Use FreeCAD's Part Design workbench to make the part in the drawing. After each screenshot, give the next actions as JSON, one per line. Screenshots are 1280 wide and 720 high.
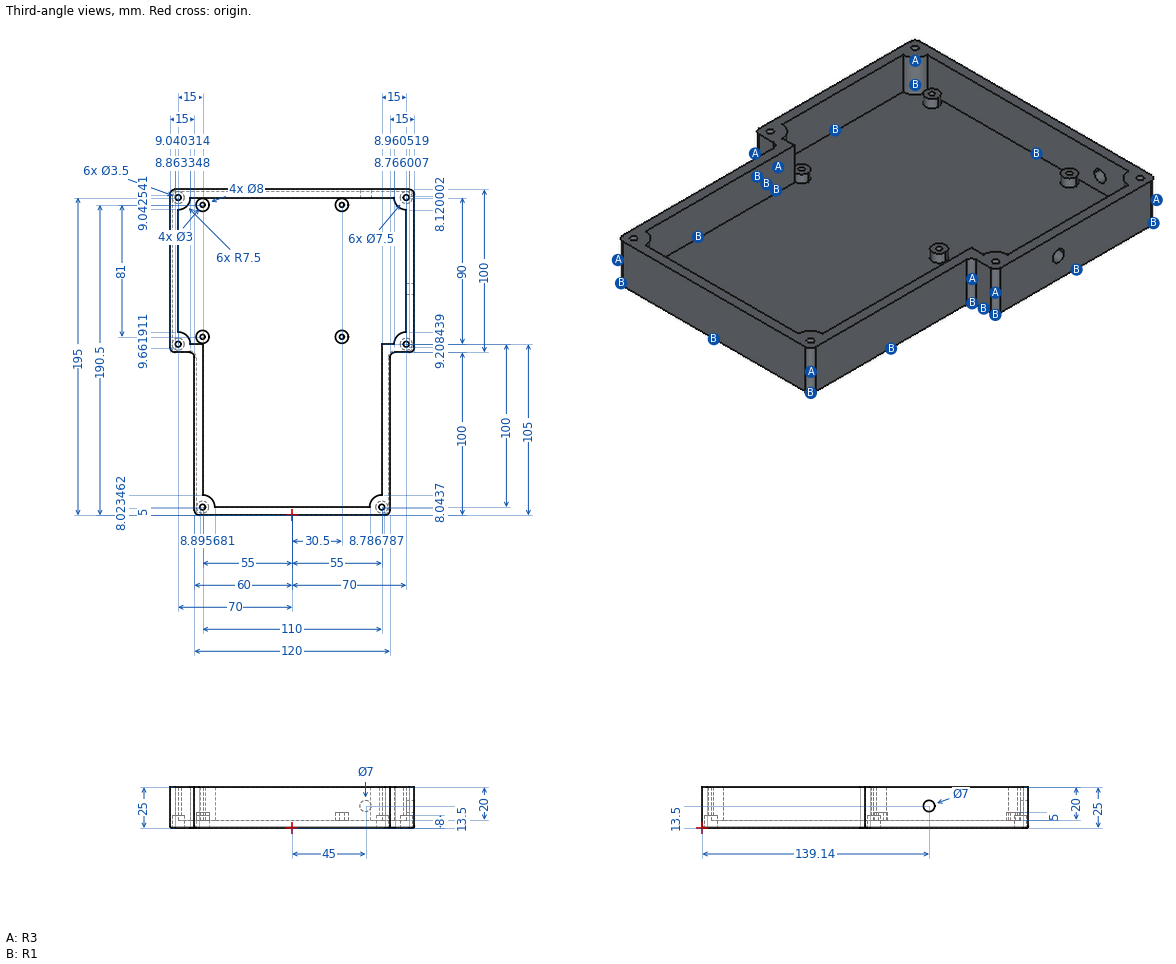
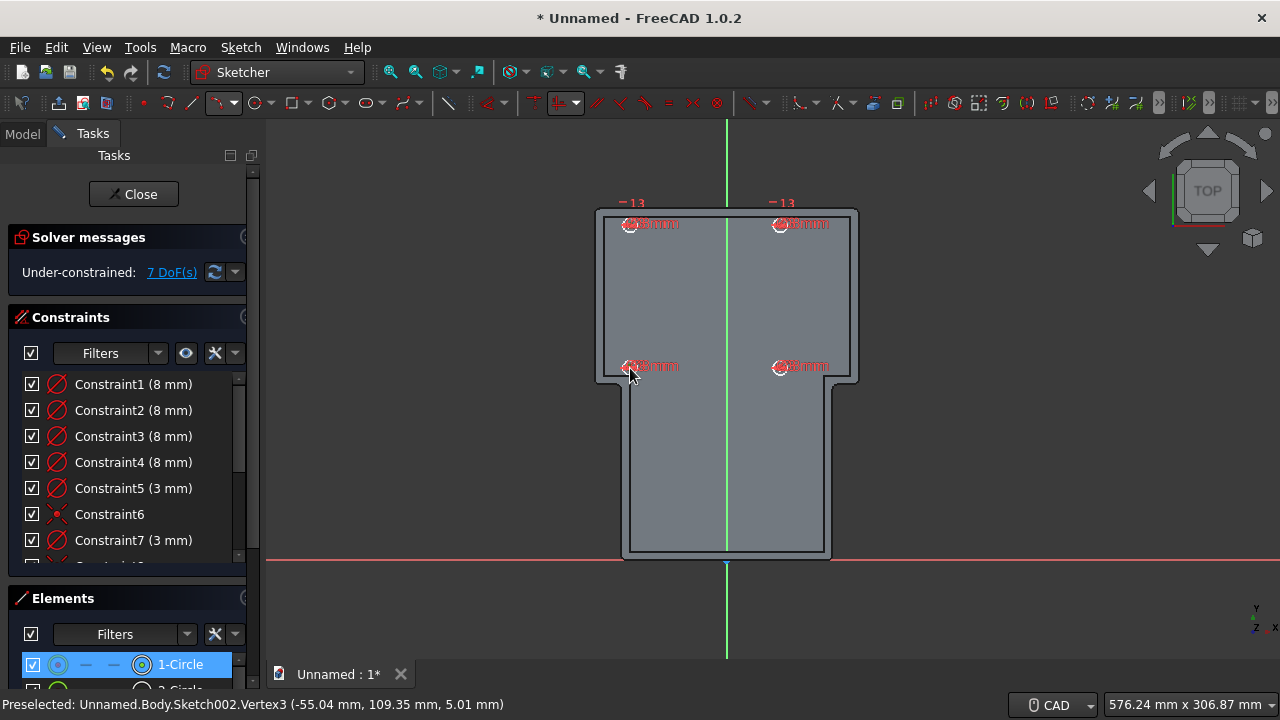
{"action": "key", "text": "v"}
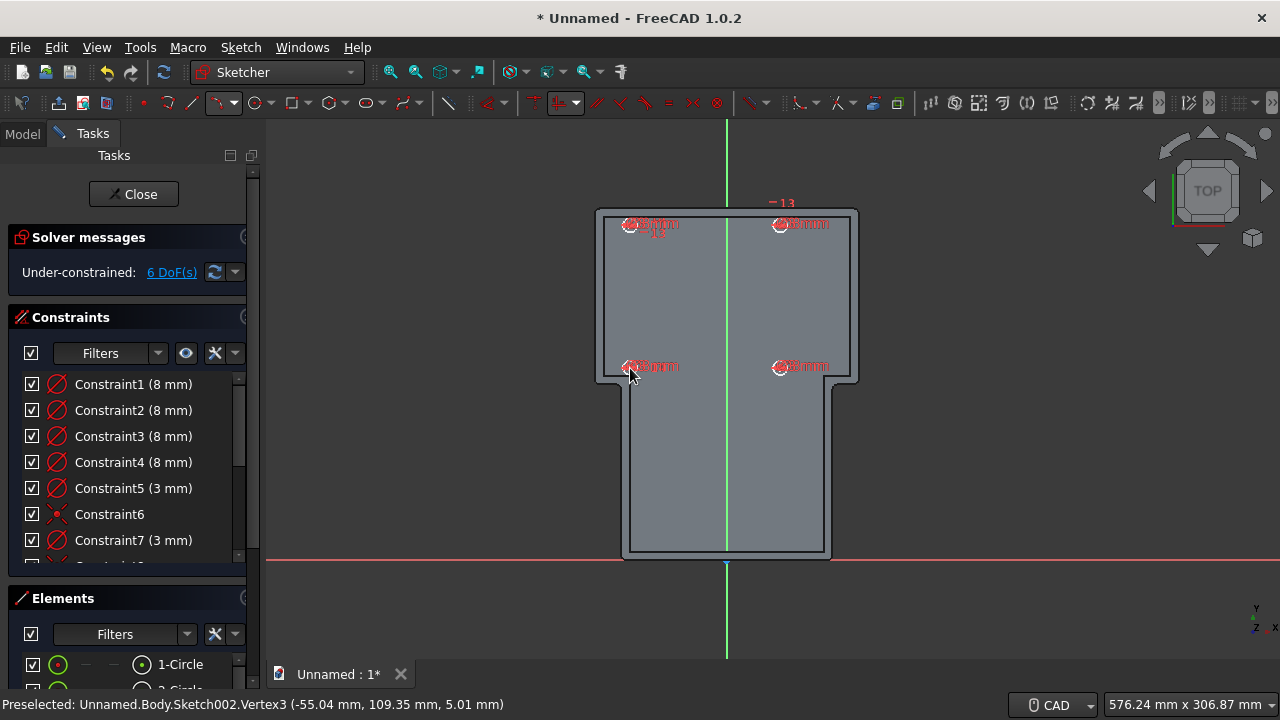
{"action": "left_click", "coordinate": [780, 225]}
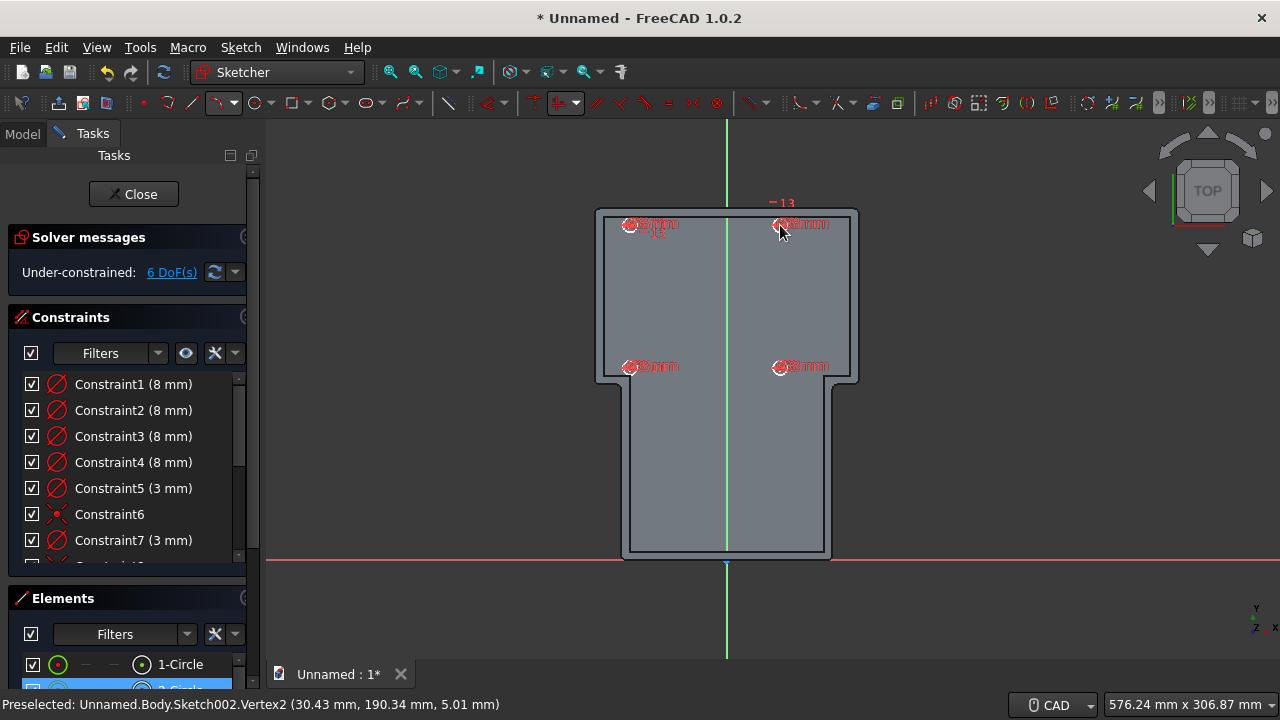
{"action": "left_click", "coordinate": [780, 368]}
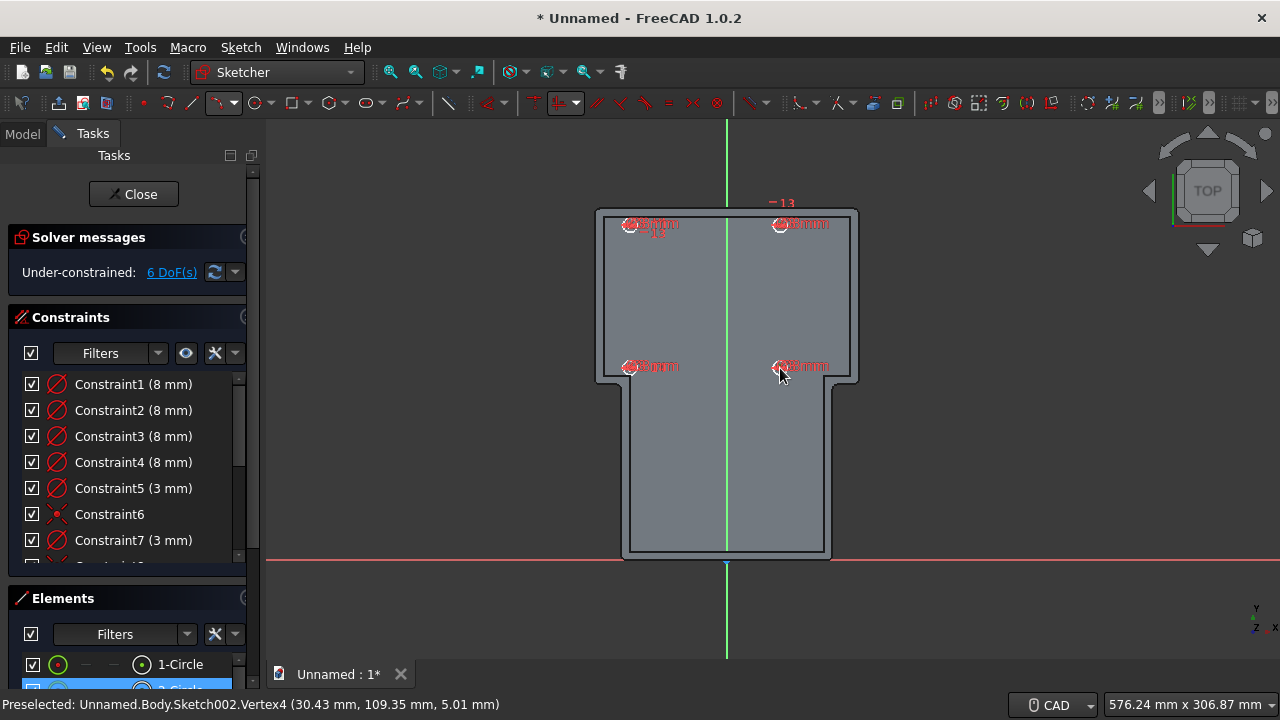
{"action": "key", "text": "v"}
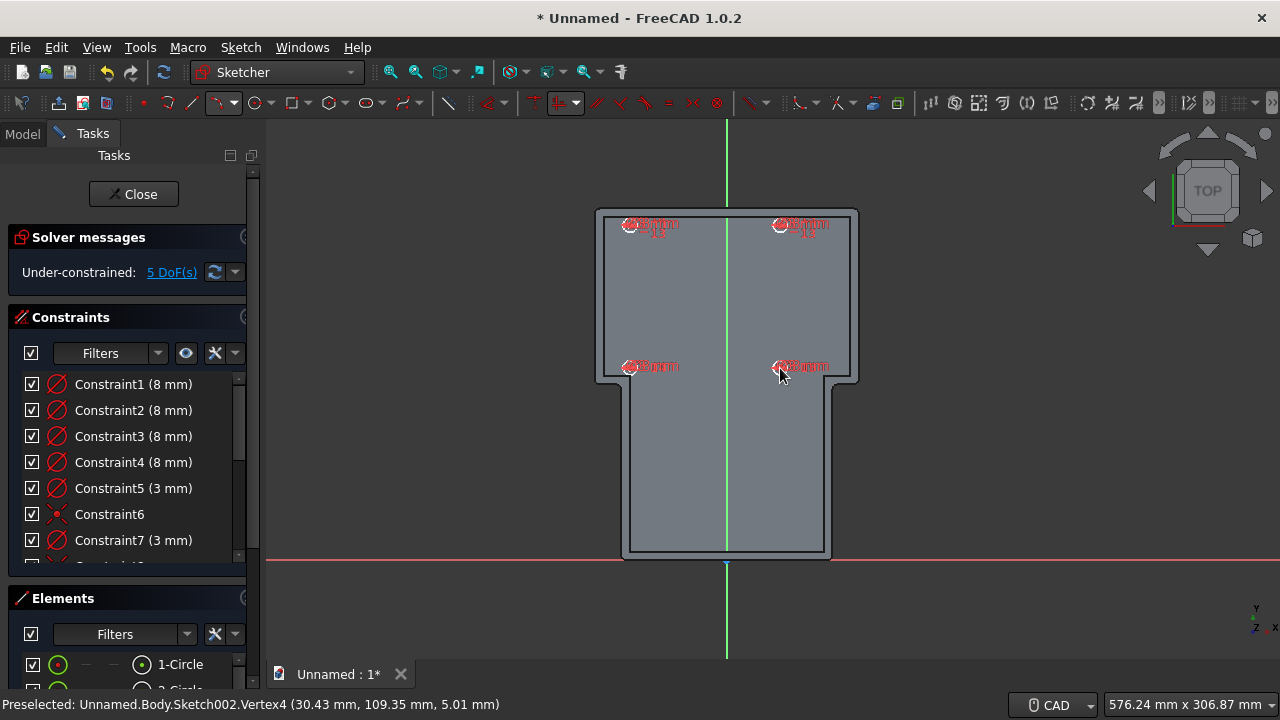
{"action": "left_click", "coordinate": [630, 368]}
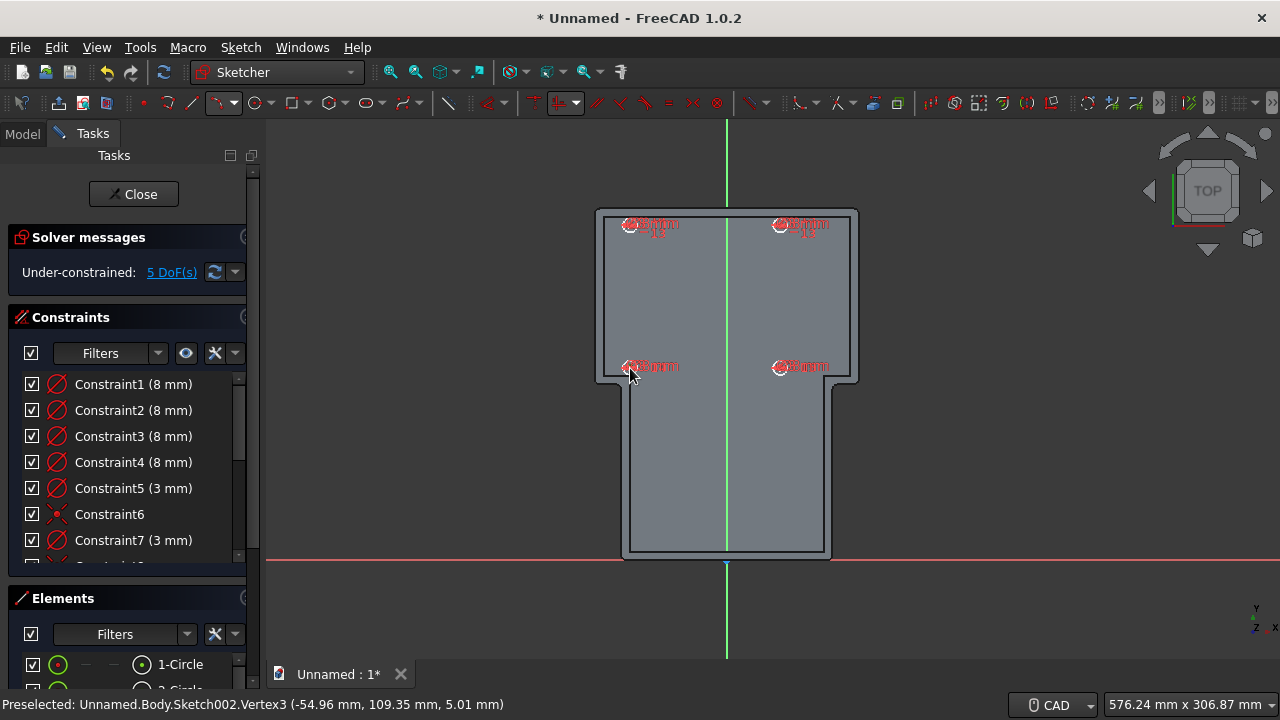
{"action": "left_click", "coordinate": [780, 368]}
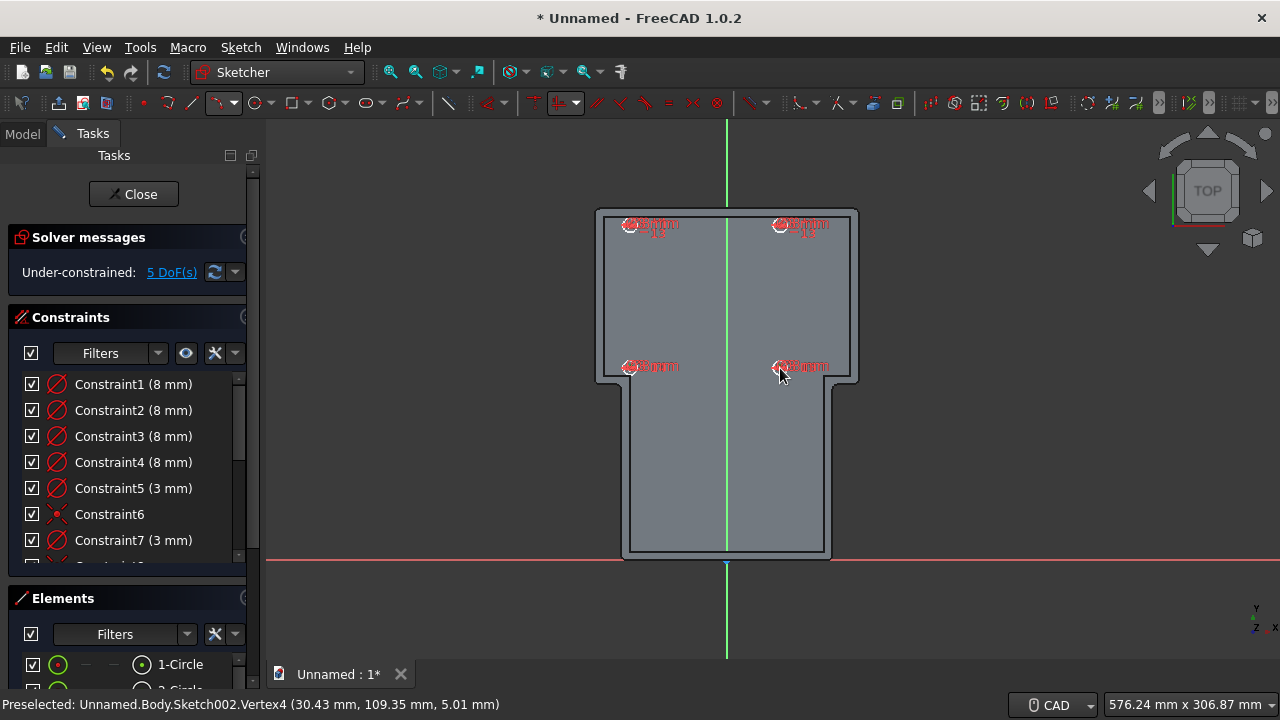
{"action": "key", "text": "h"}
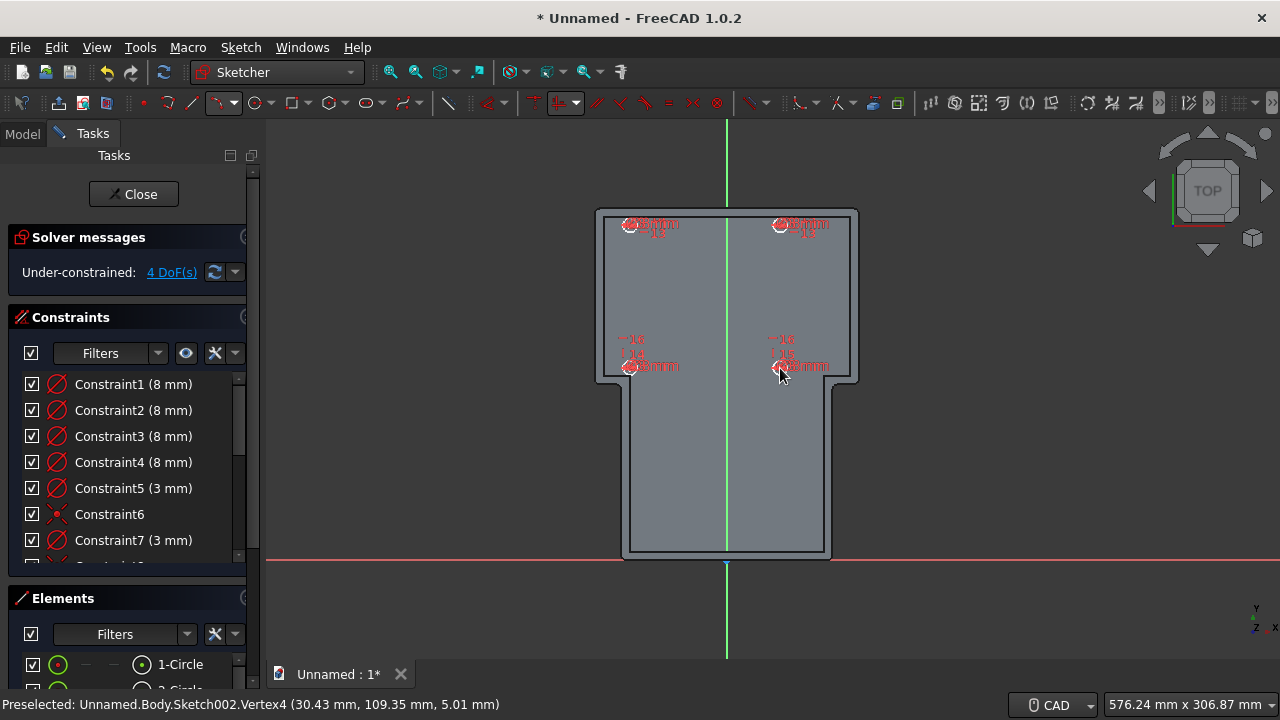
{"action": "key", "text": "d"}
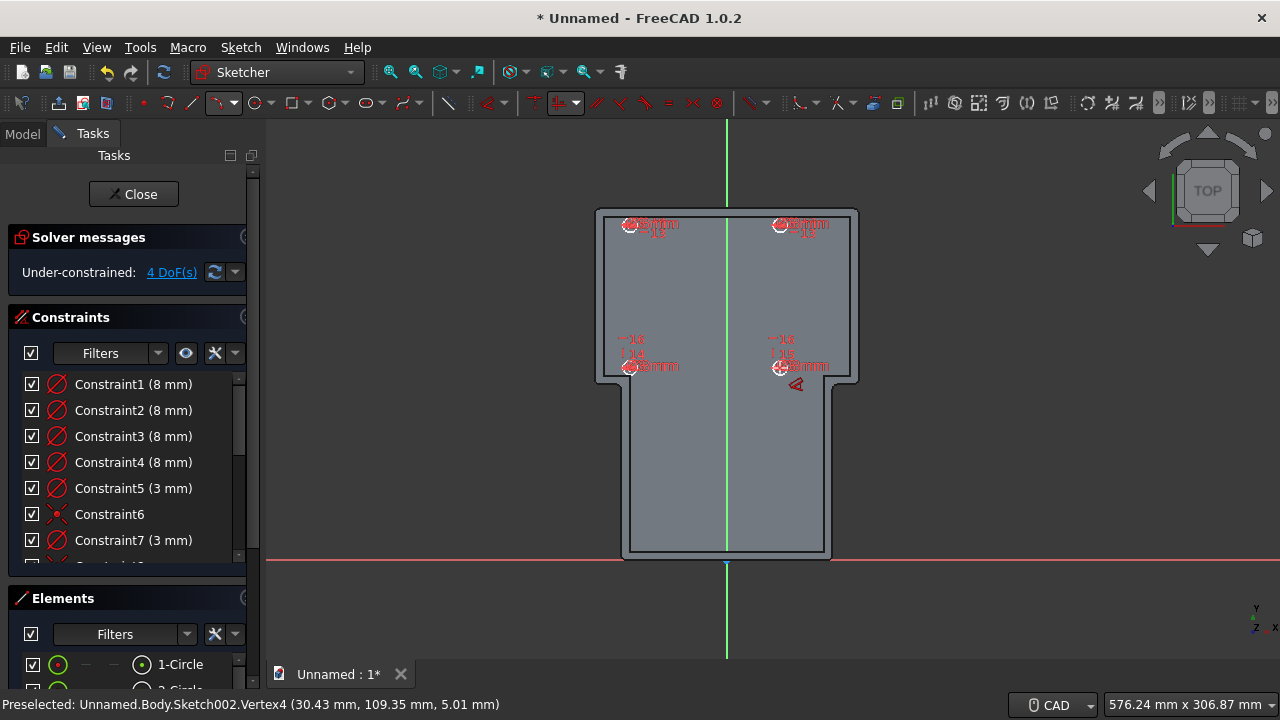
{"action": "left_click", "coordinate": [630, 225]}
{"action": "left_click", "coordinate": [678, 594]}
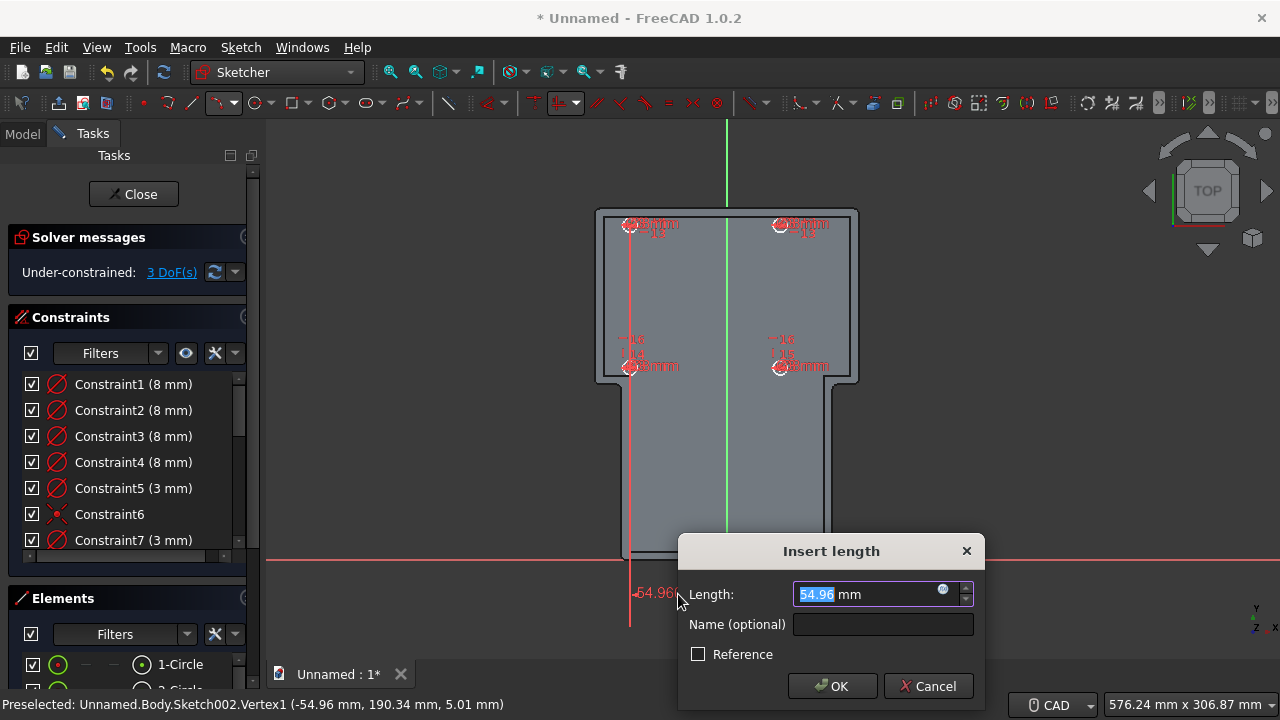
{"action": "type", "text": "55"}
{"action": "key", "text": "Return"}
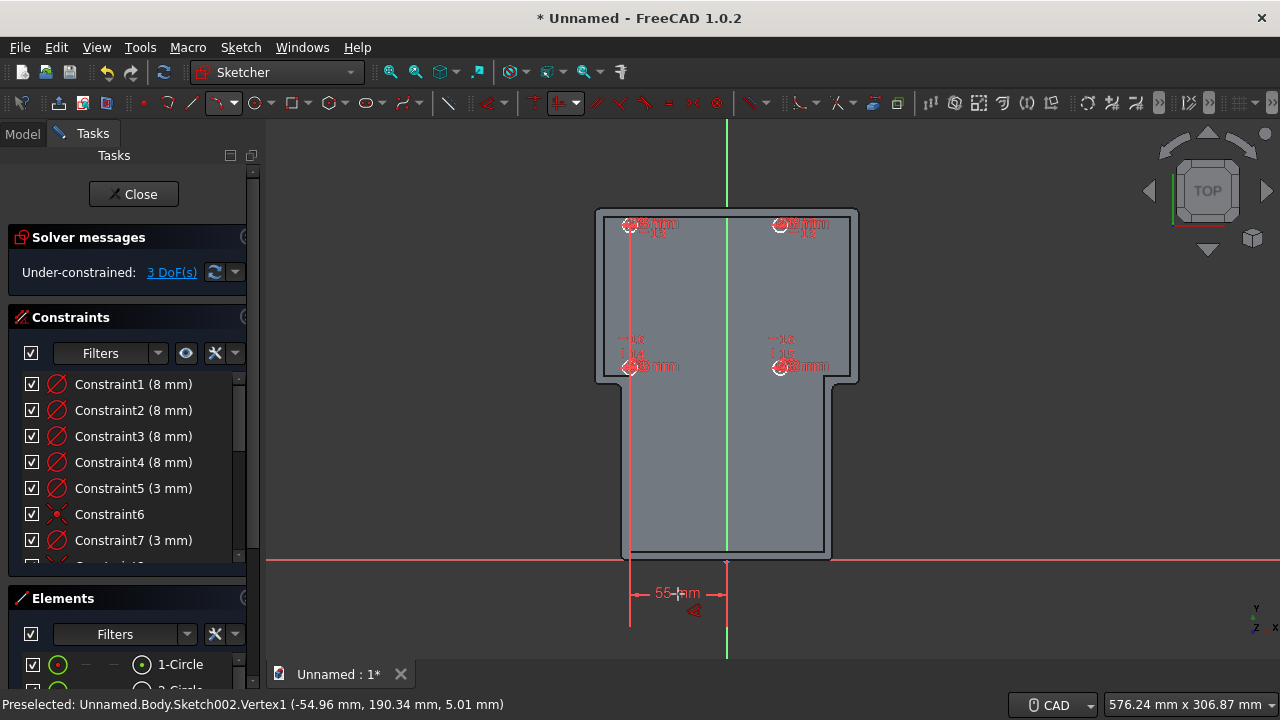
{"action": "left_click", "coordinate": [630, 225]}